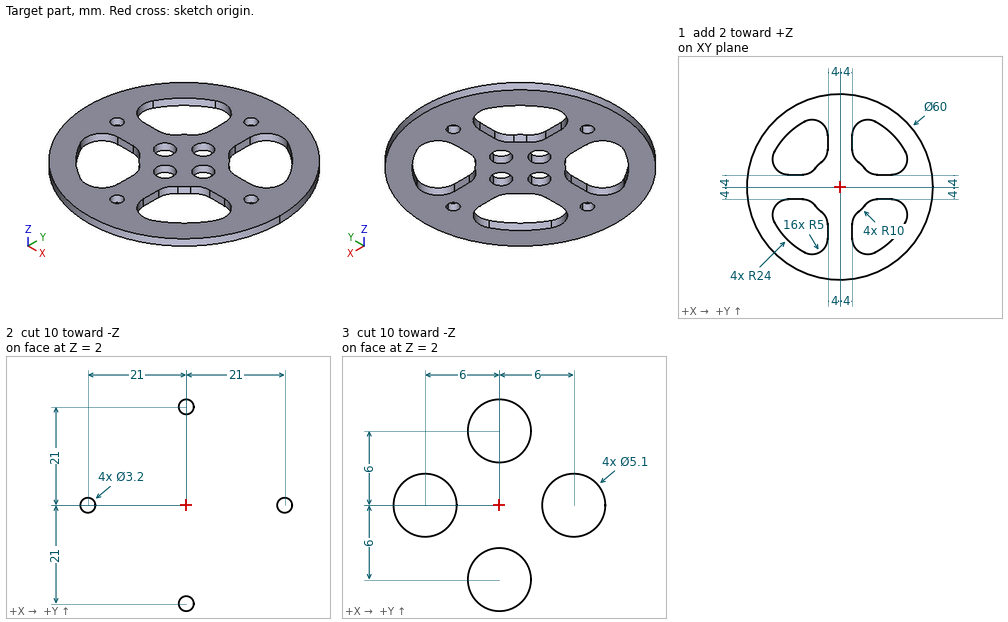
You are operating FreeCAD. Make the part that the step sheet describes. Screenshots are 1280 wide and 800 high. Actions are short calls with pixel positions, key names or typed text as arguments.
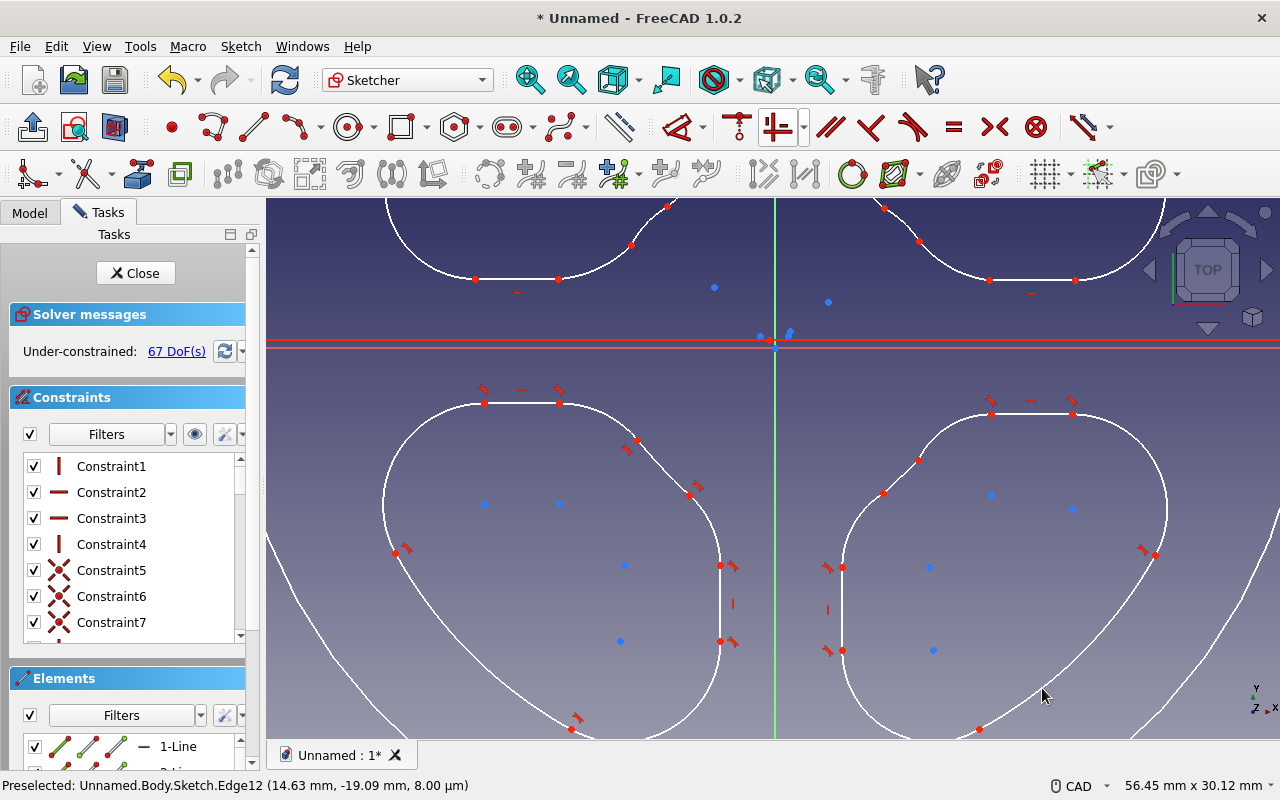
click(1042, 688)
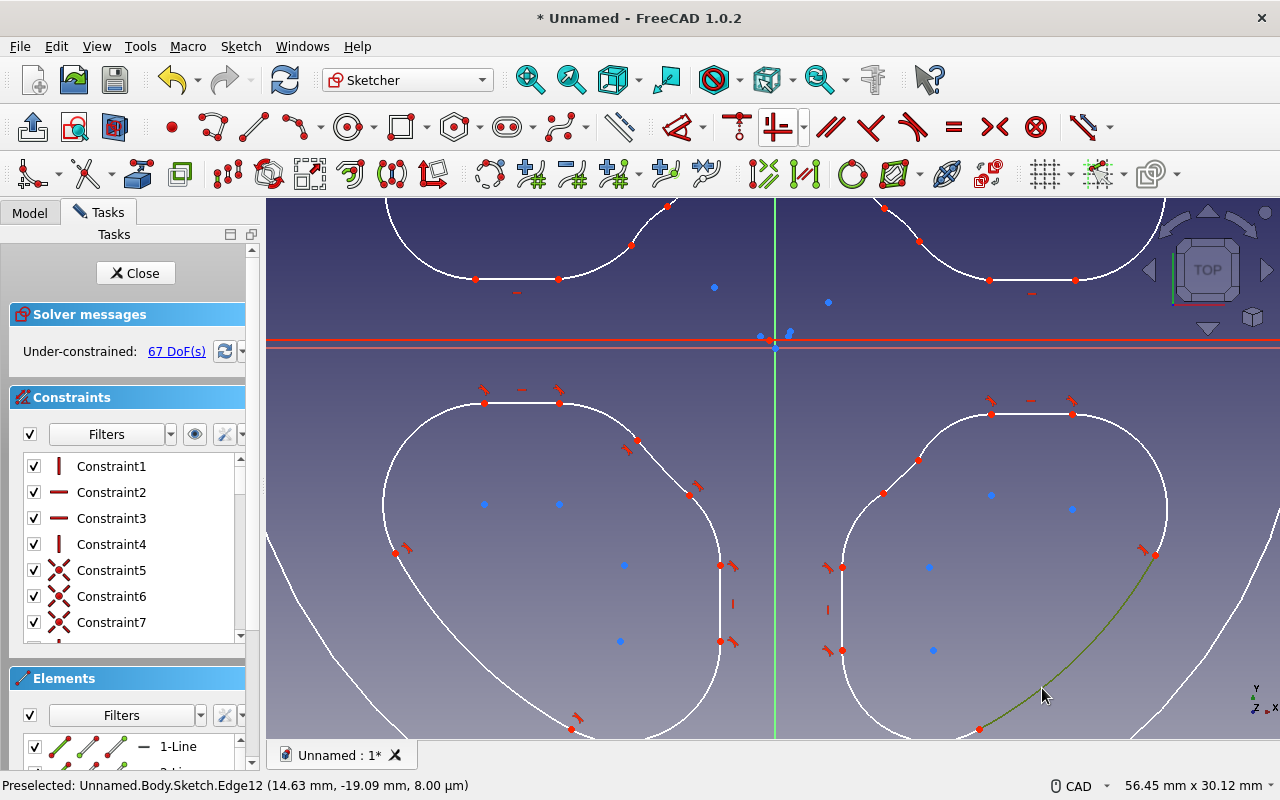
click(860, 704)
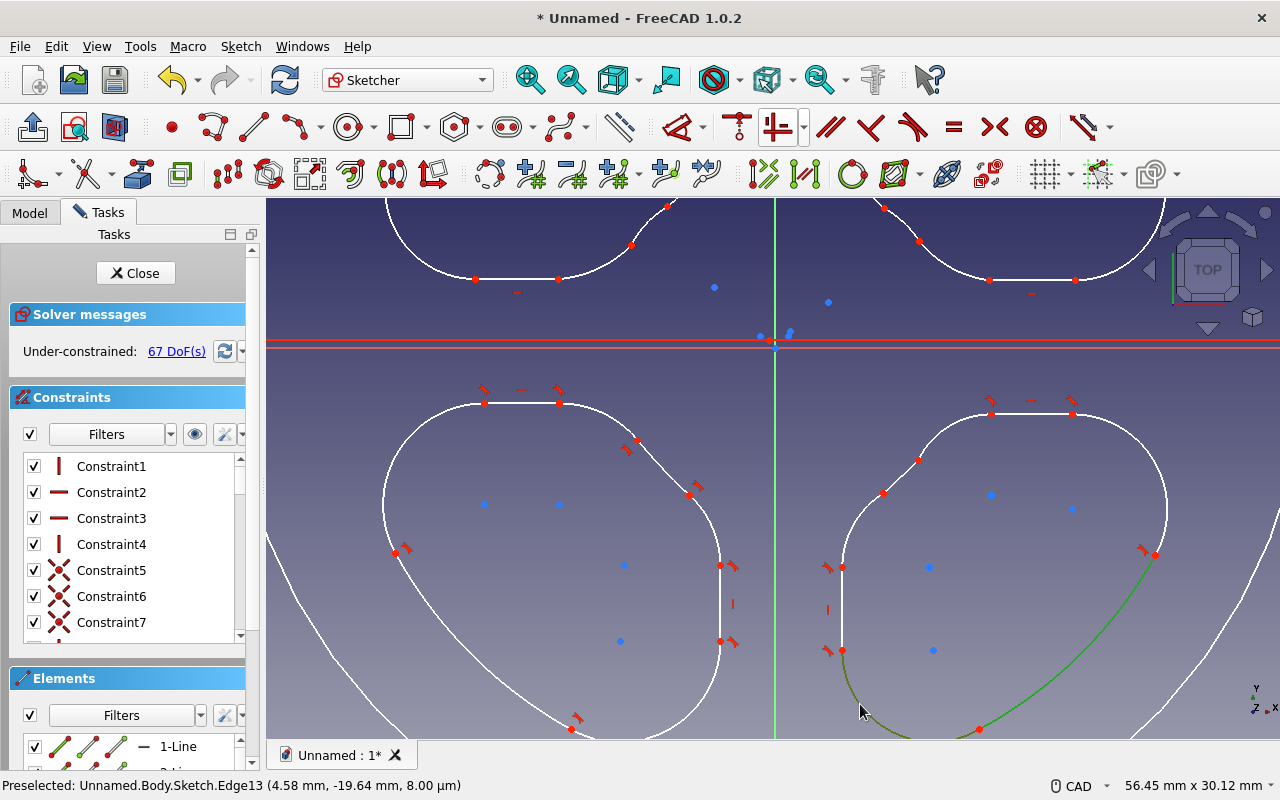
click(913, 128)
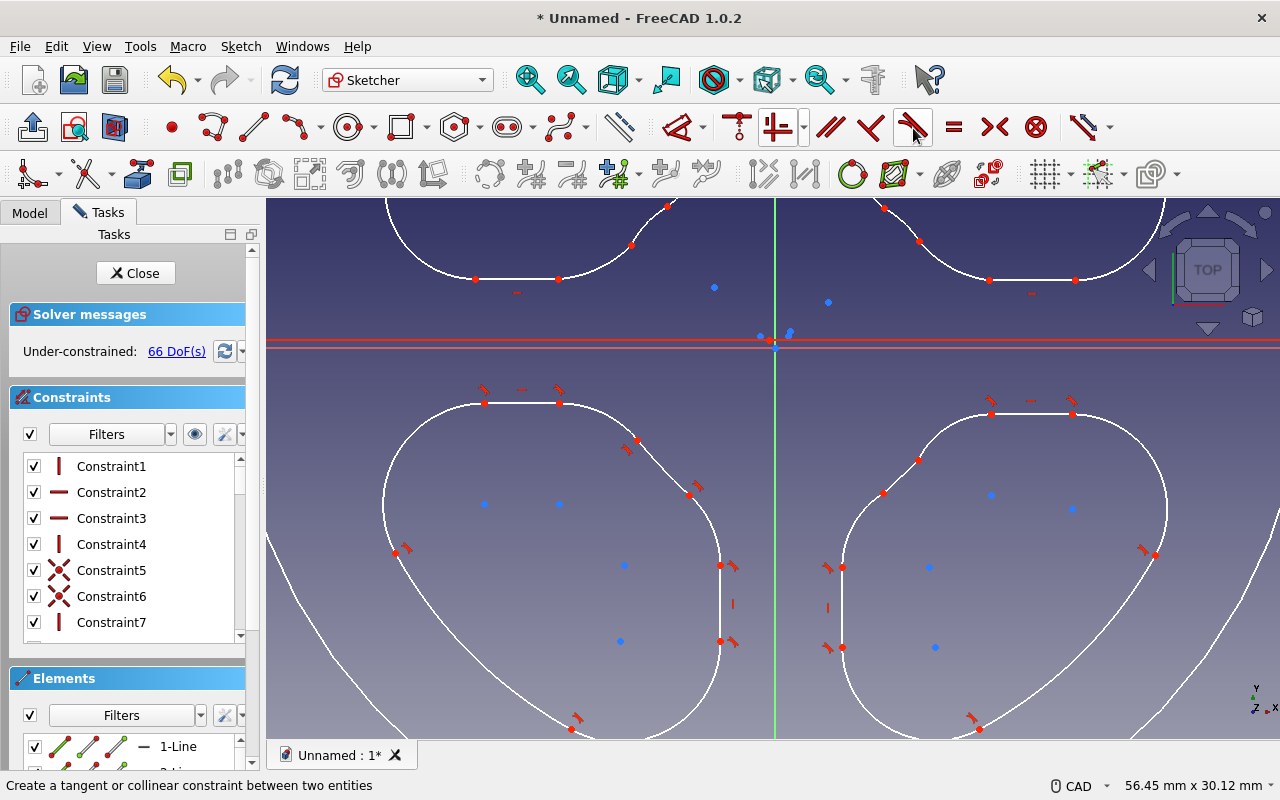
click(863, 511)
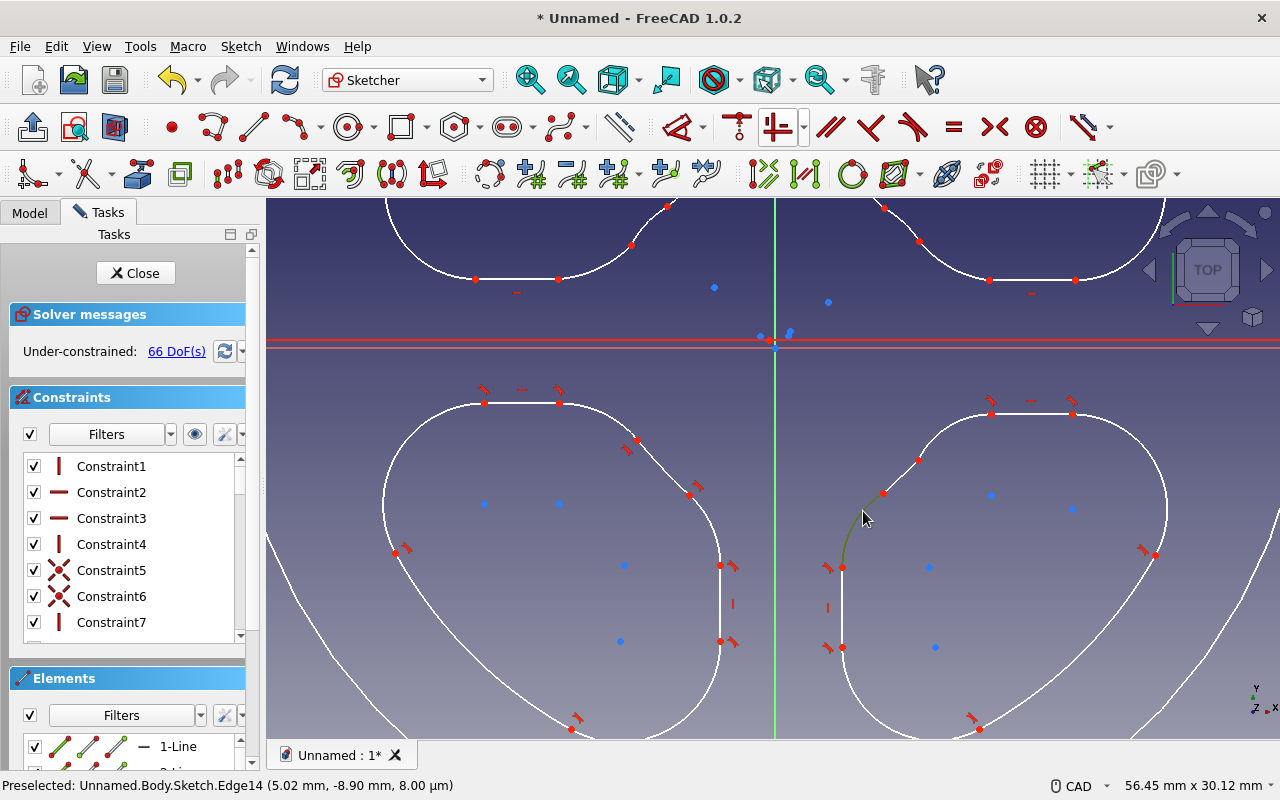
click(894, 484)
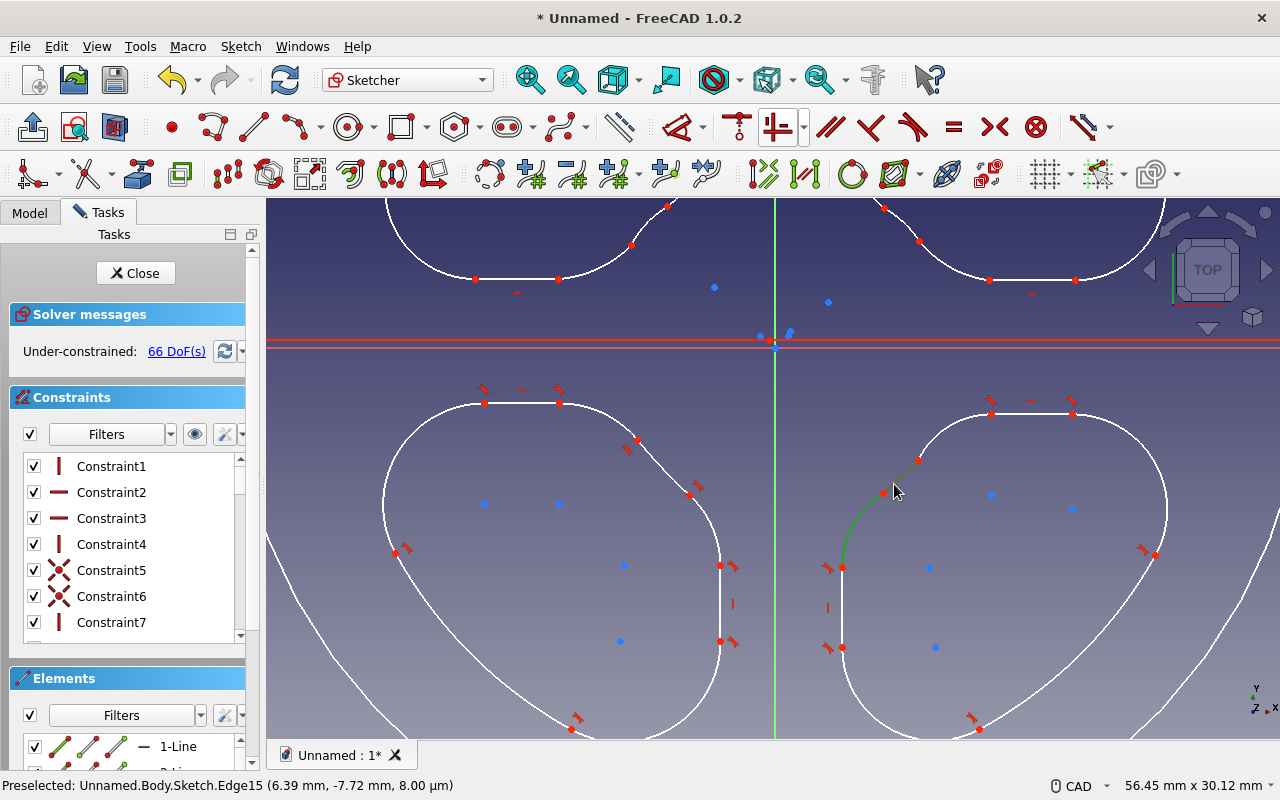
click(913, 128)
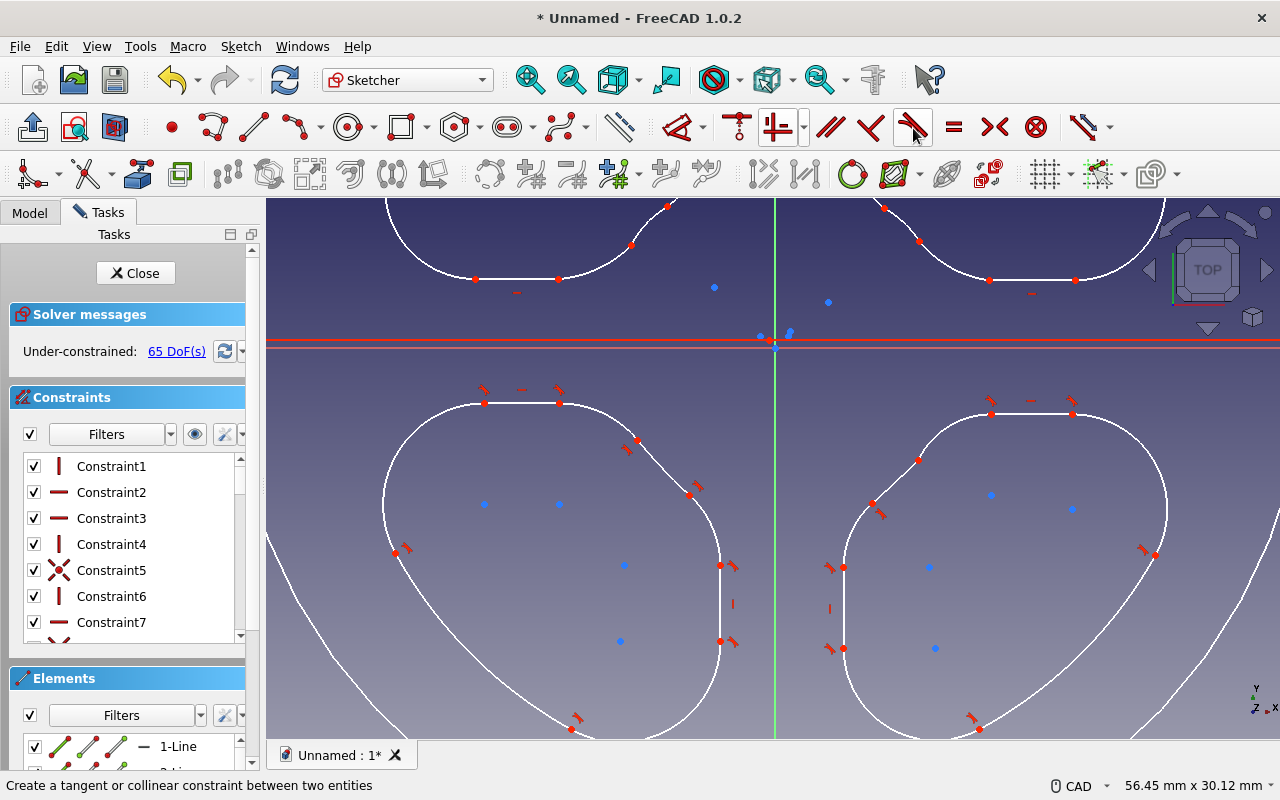
click(886, 491)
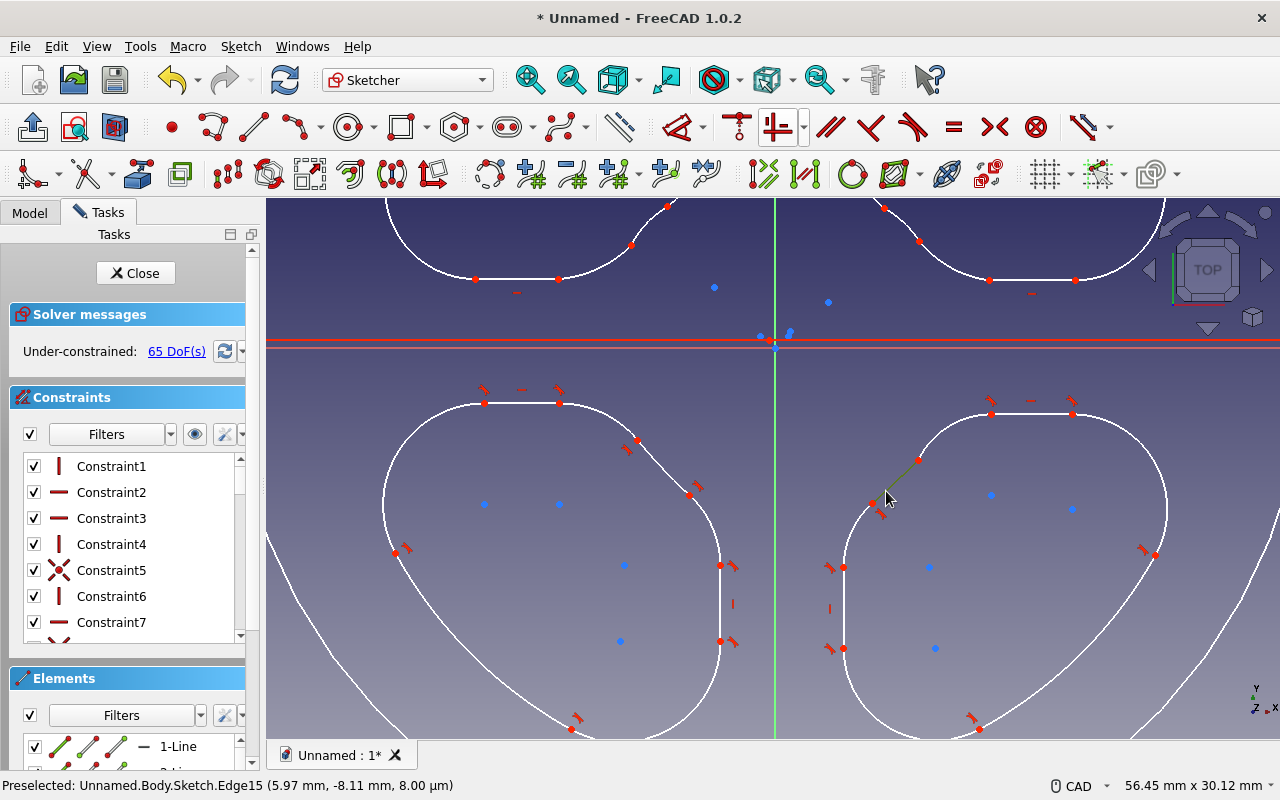
click(964, 419)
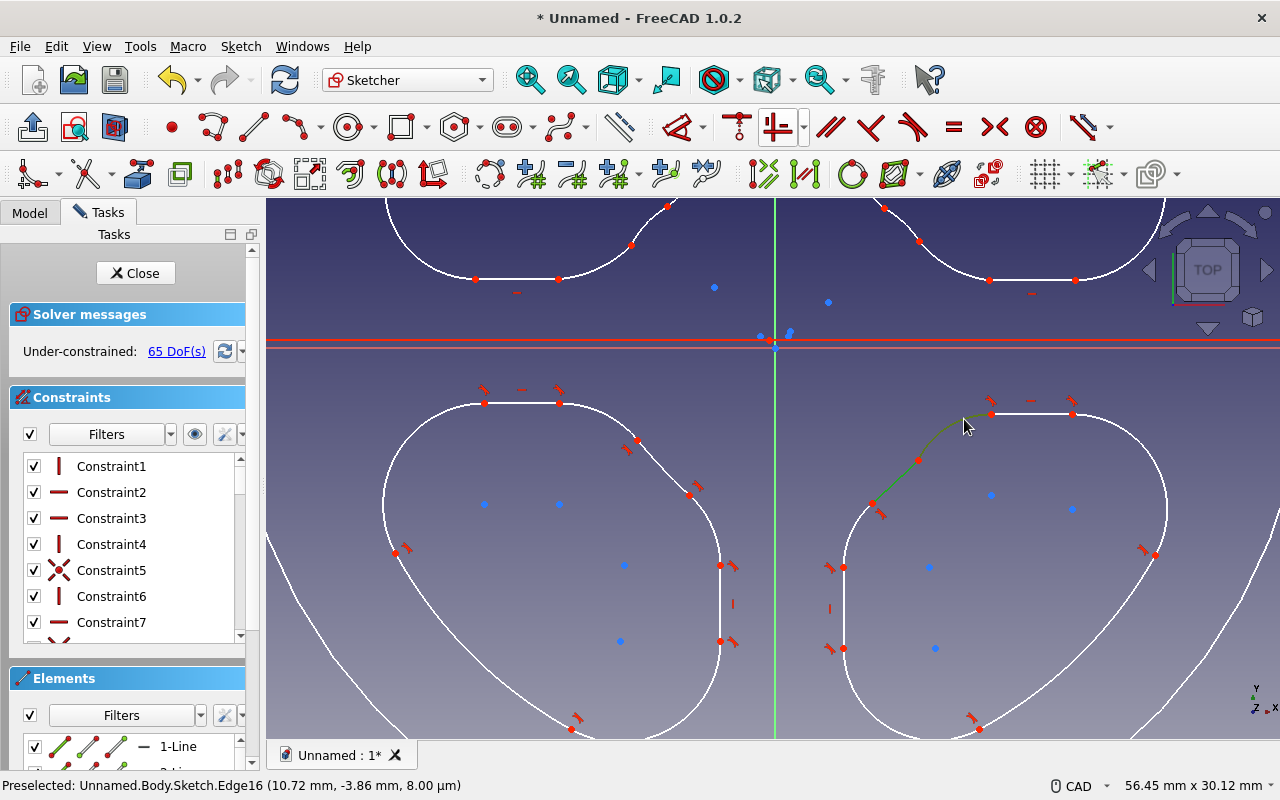
click(913, 128)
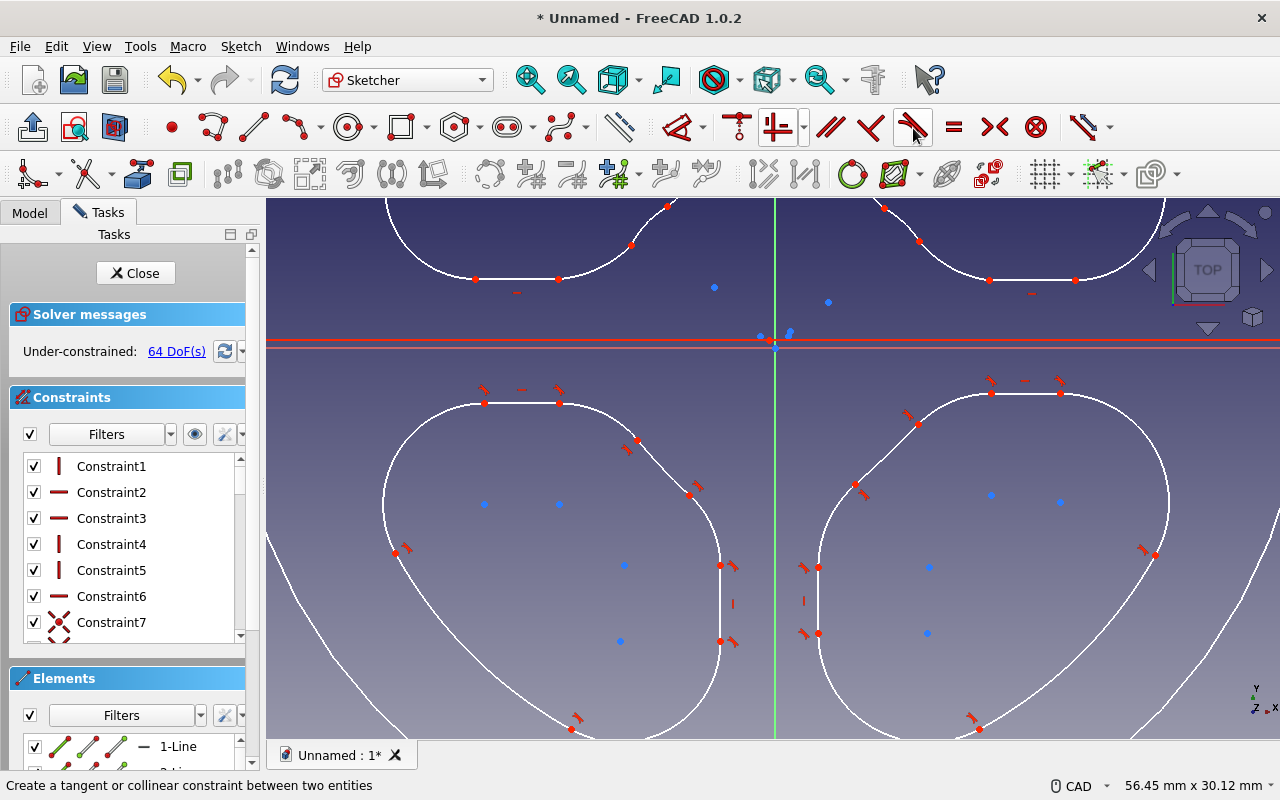
scroll(674, 520, down, 6)